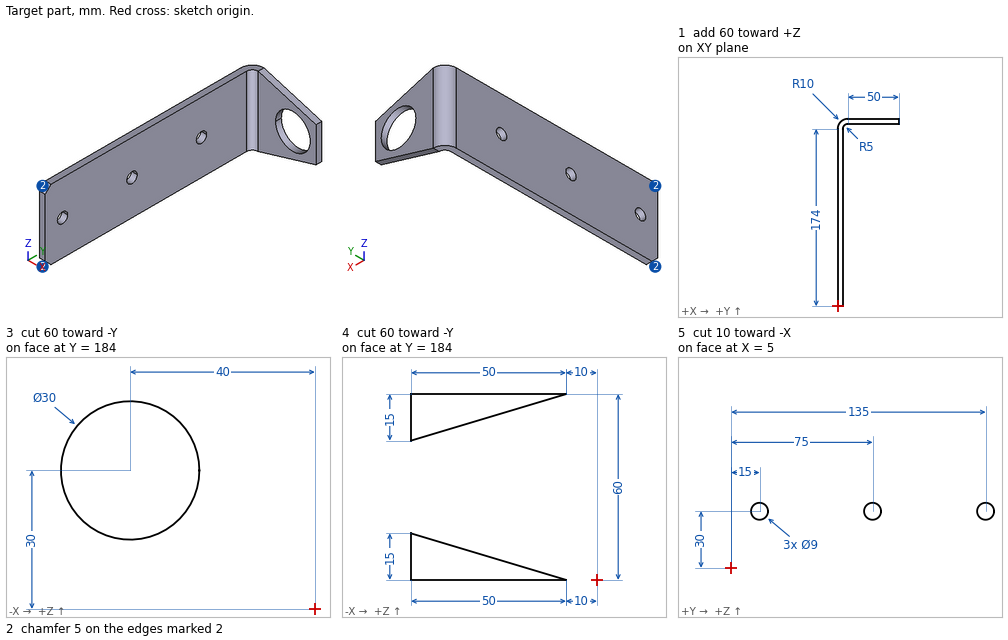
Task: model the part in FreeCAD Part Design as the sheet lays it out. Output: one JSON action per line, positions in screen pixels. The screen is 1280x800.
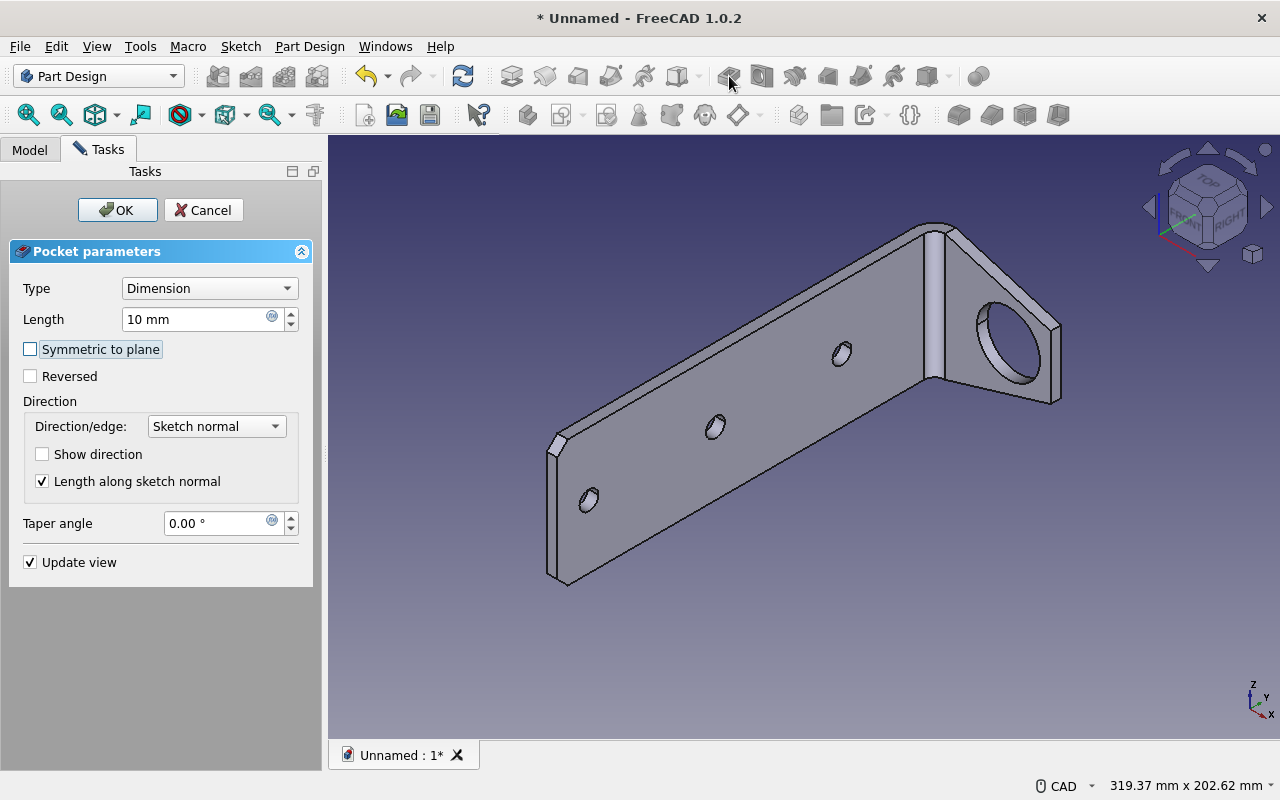
{"action": "left_click", "coordinate": [118, 210]}